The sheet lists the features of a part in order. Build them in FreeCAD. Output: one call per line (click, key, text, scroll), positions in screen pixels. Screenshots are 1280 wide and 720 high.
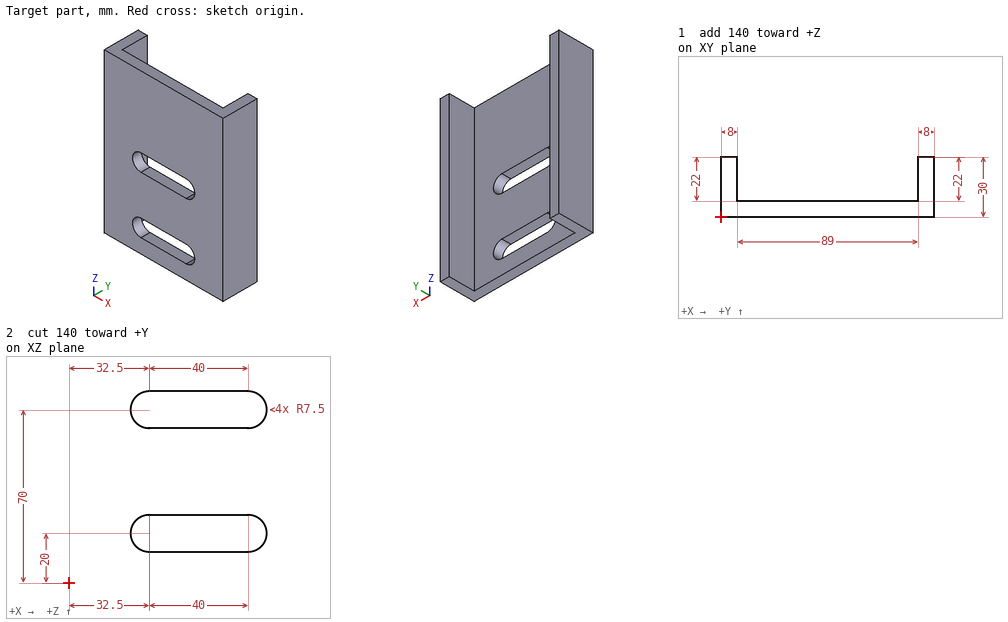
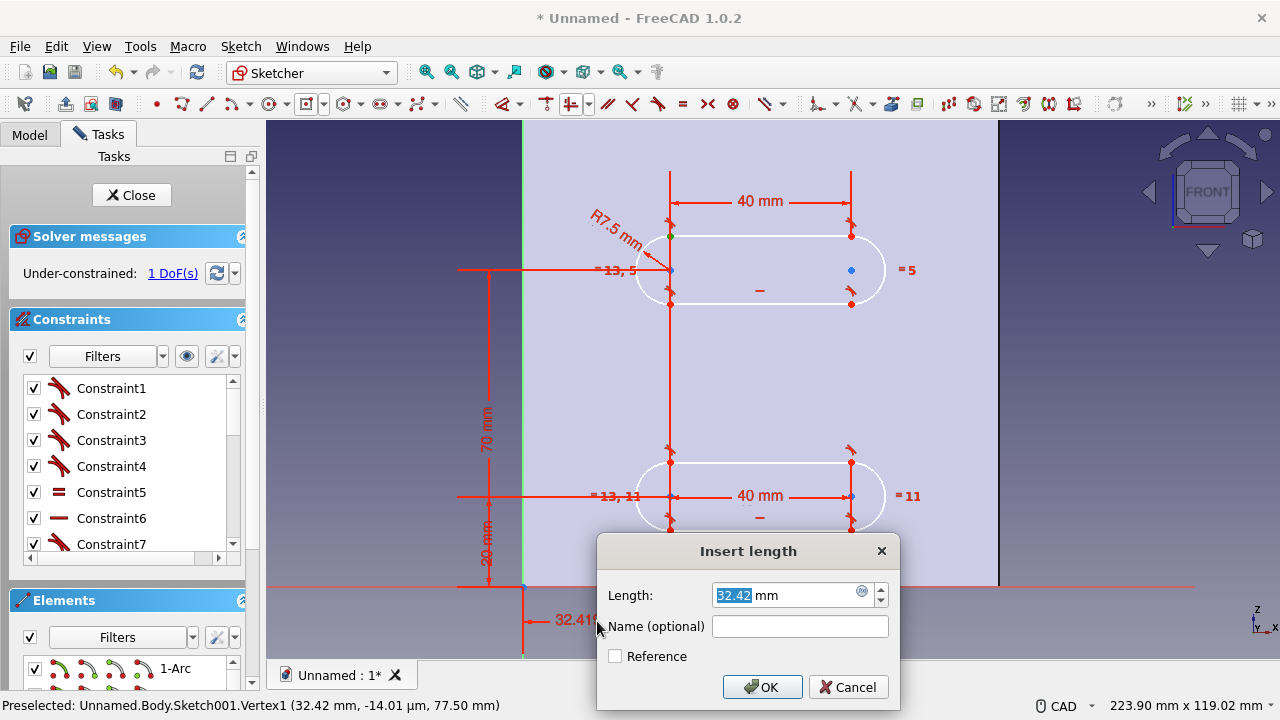
text(32.5)
key(Return)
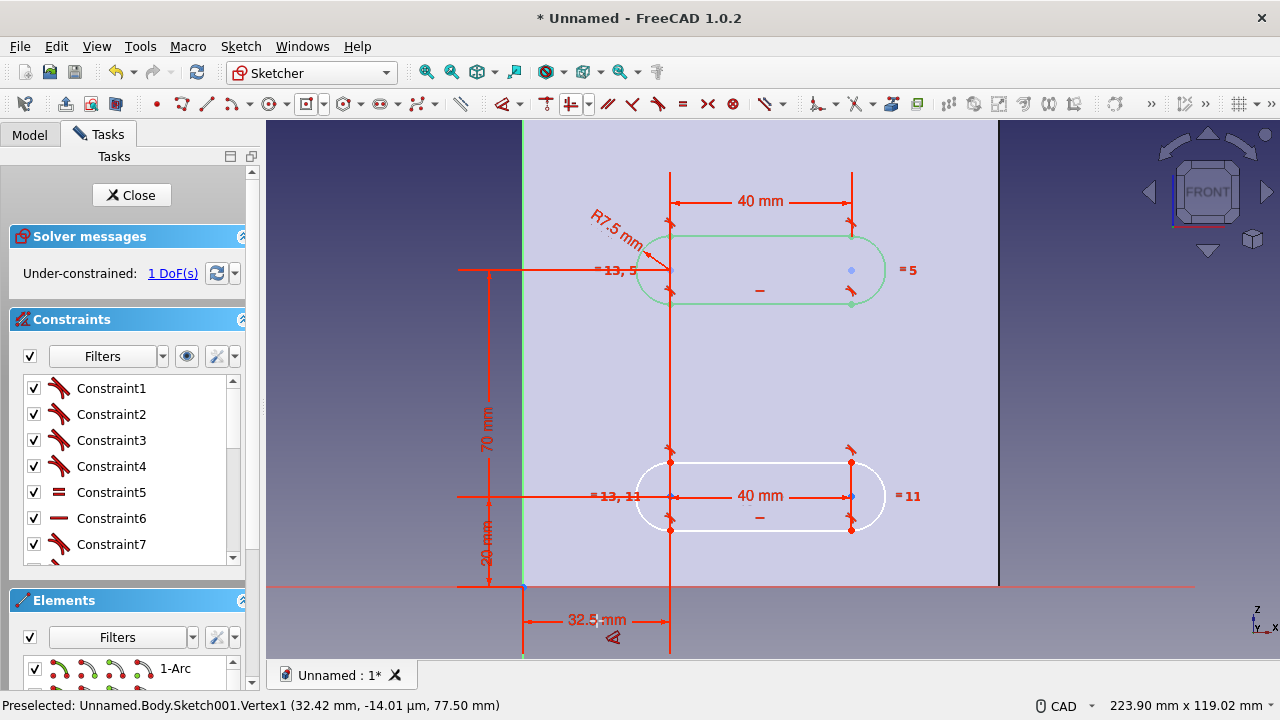
click(670, 463)
click(597, 429)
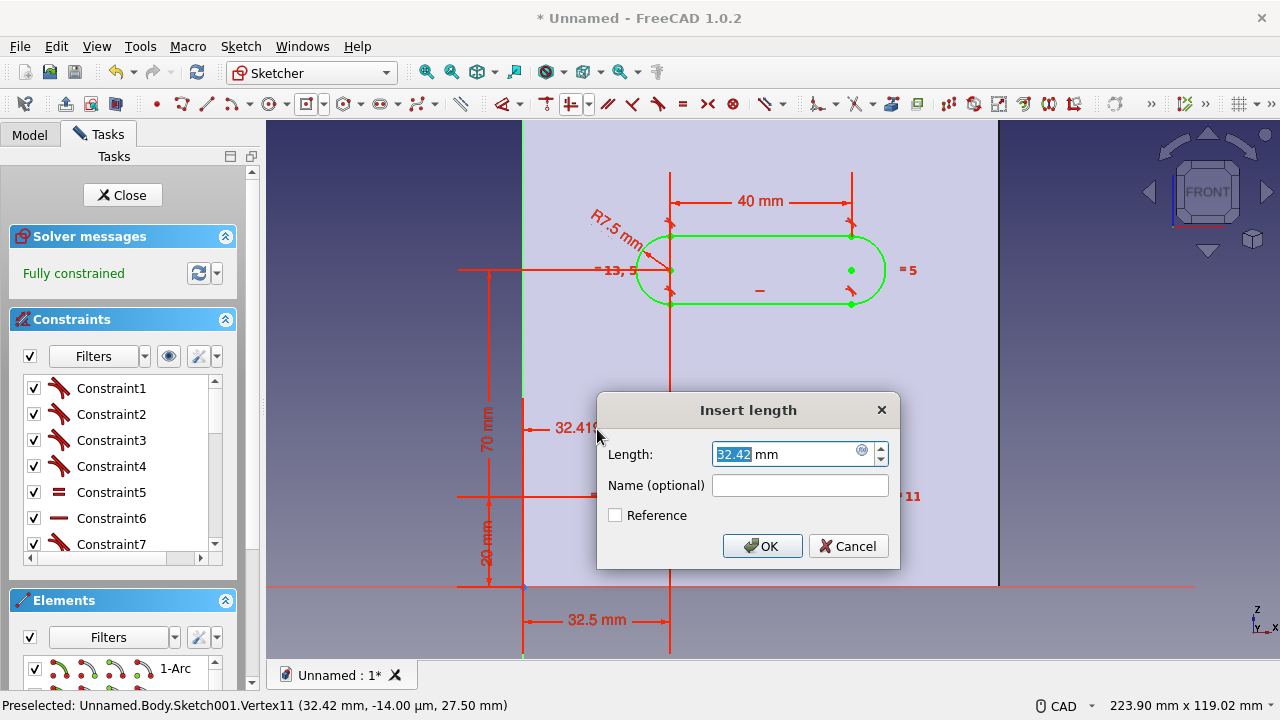
text(32.5)
key(Return)
key(Escape)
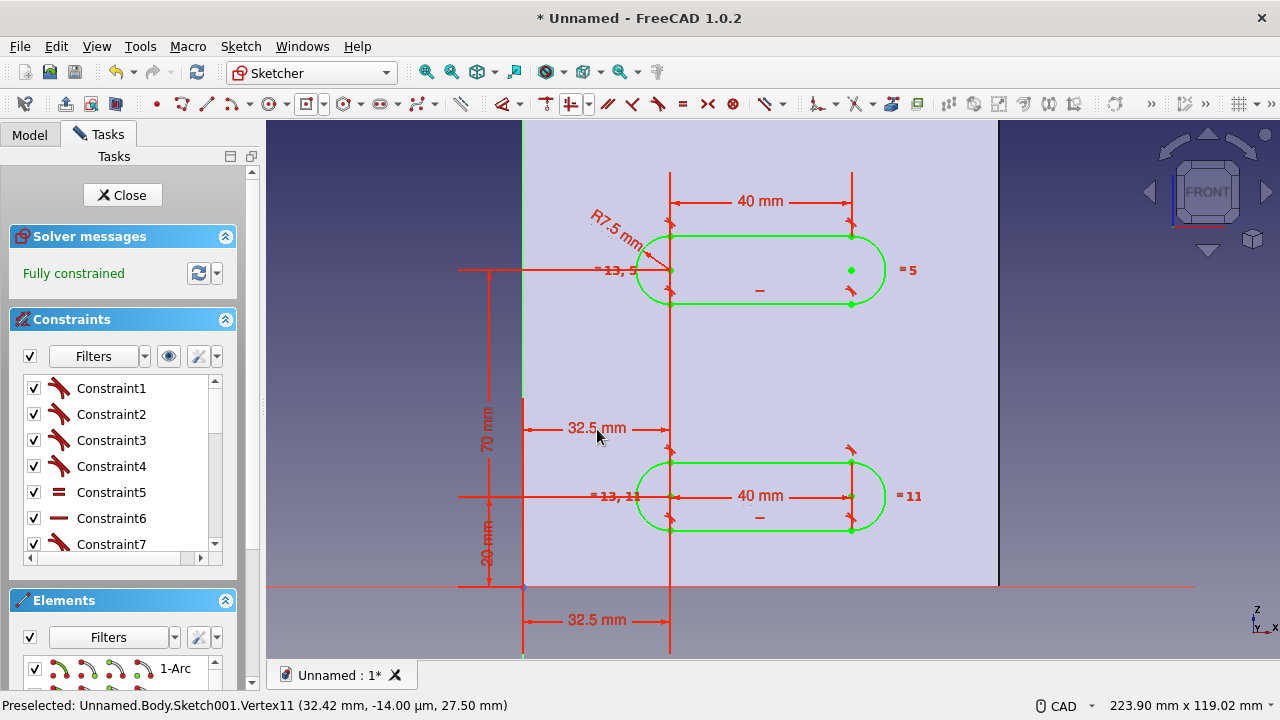
click(123, 195)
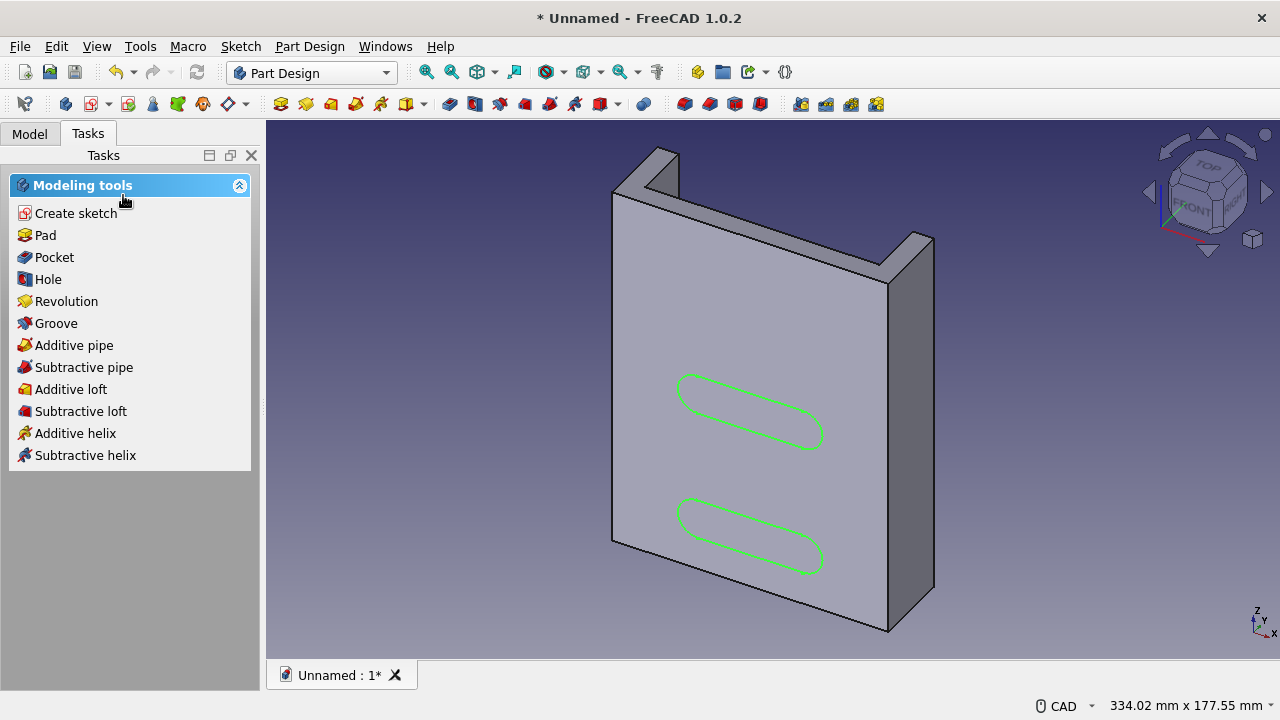
click(450, 104)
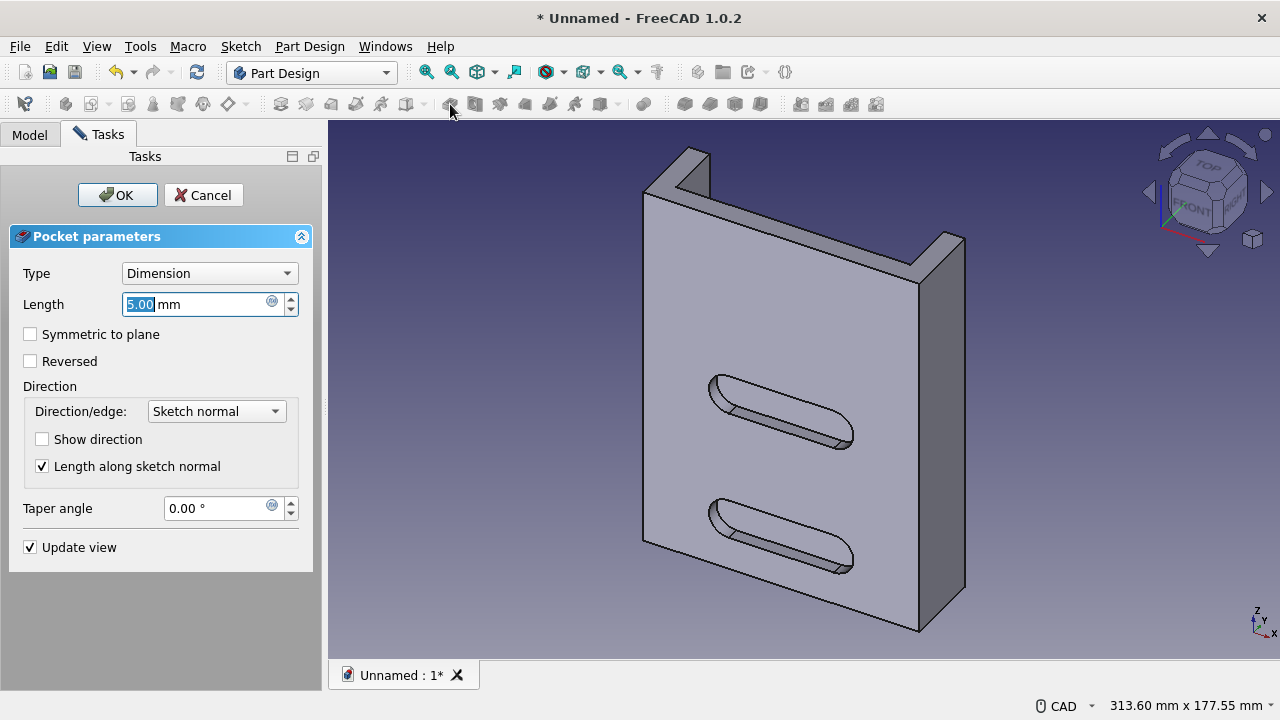
text(140)
key(Tab)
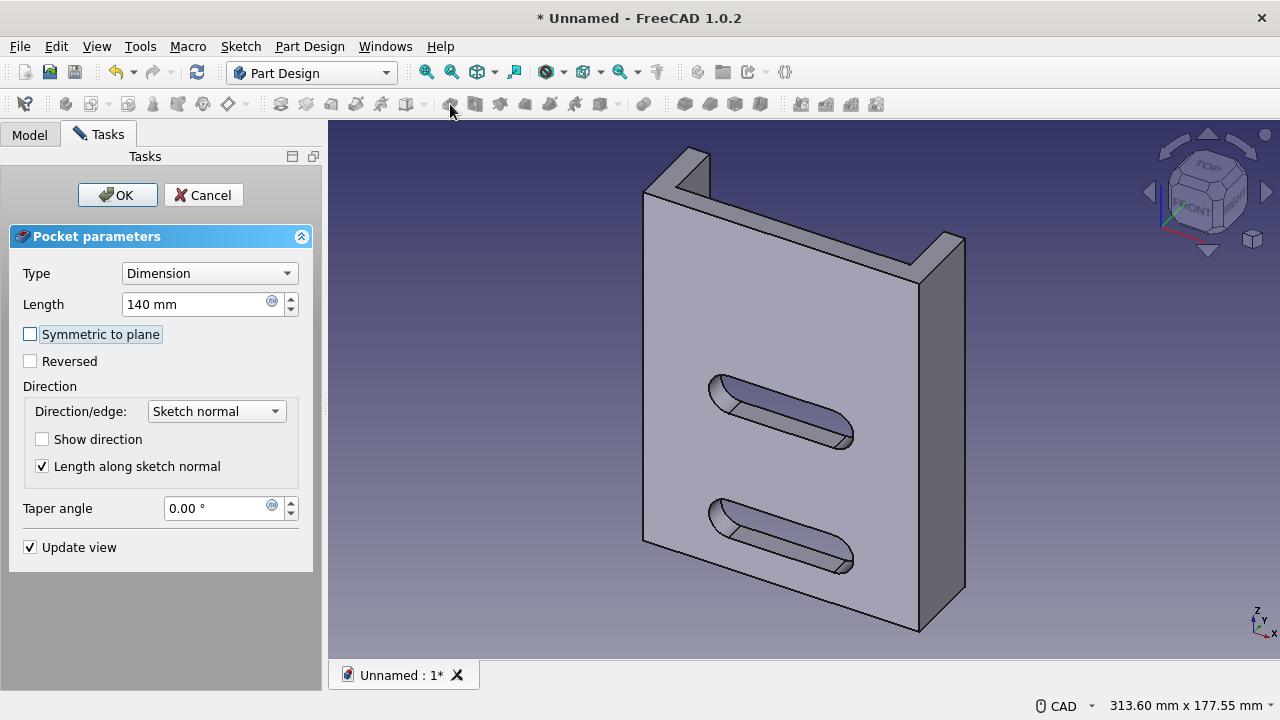
click(118, 195)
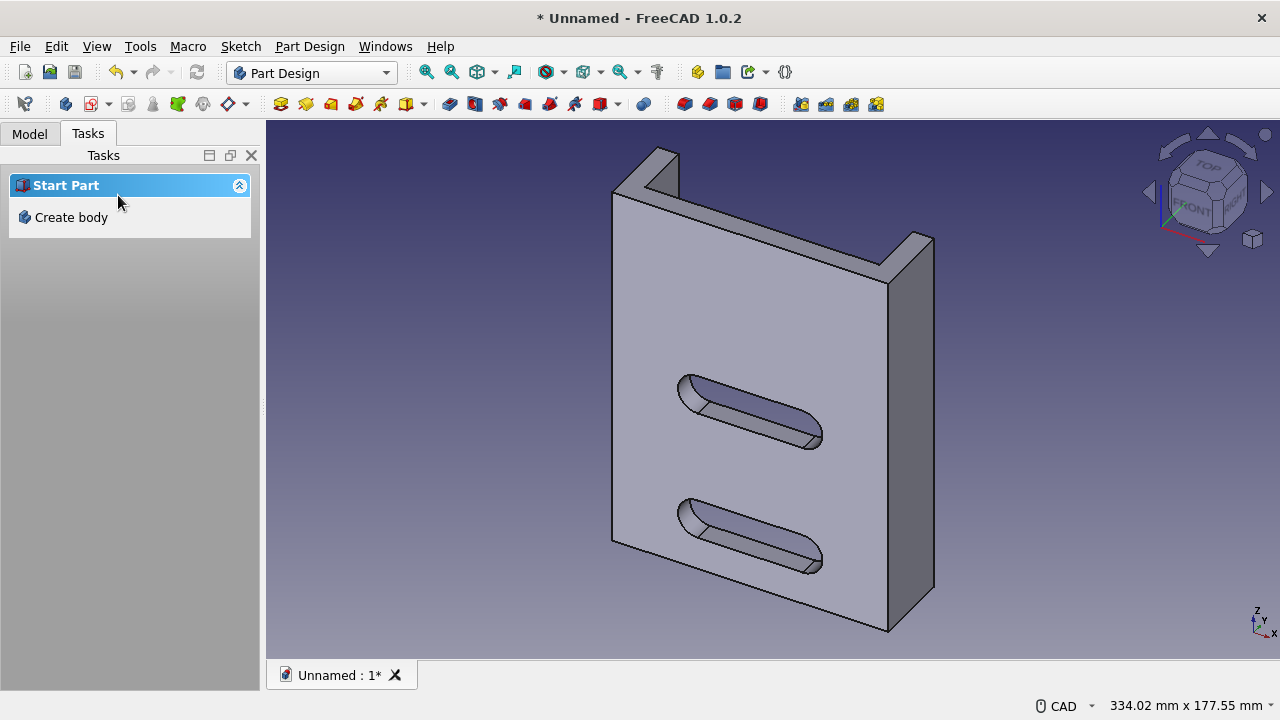
key(0)